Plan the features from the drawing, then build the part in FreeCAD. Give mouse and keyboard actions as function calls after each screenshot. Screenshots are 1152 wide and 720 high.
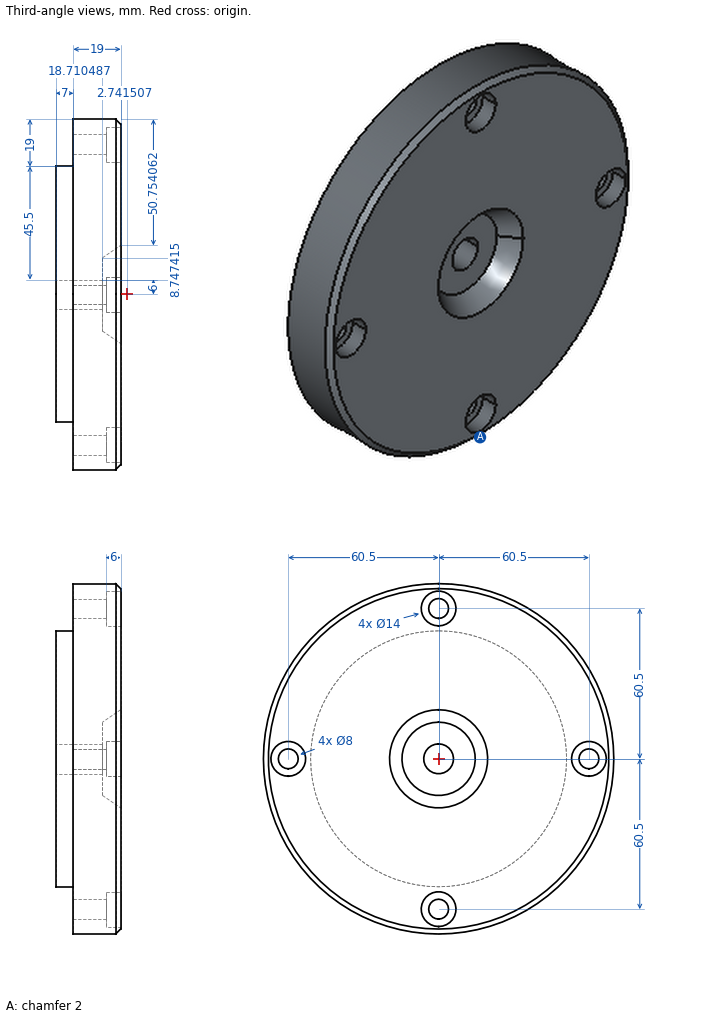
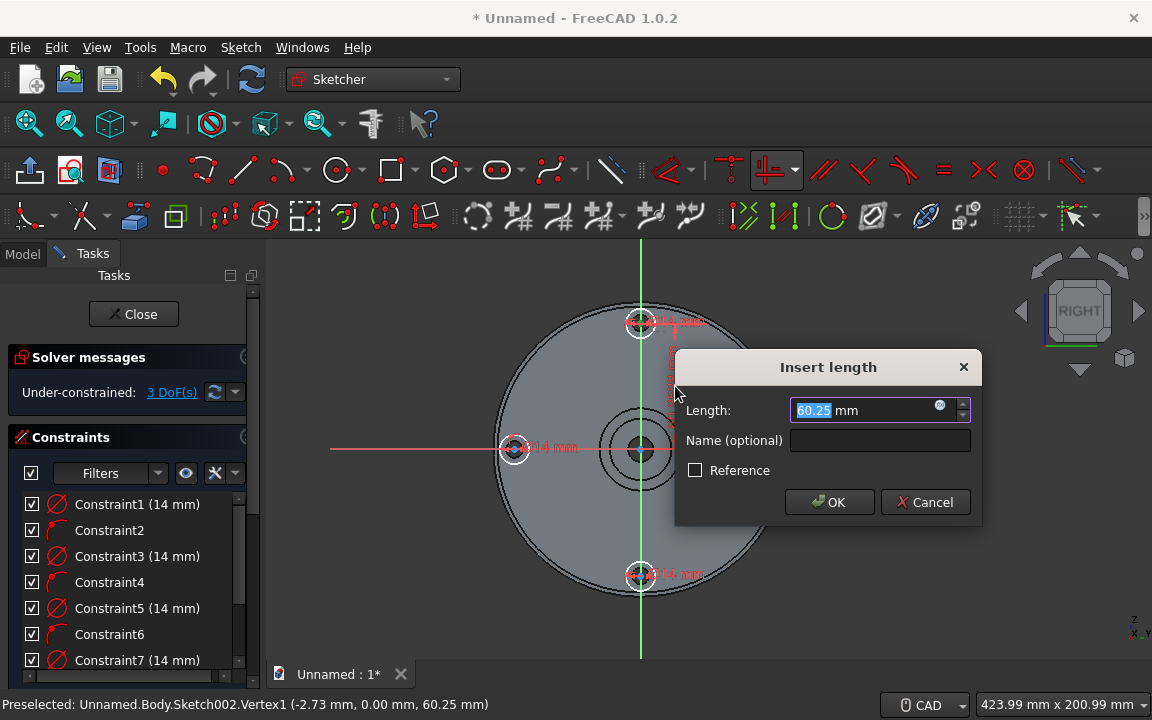
text(60.5)
key(Return)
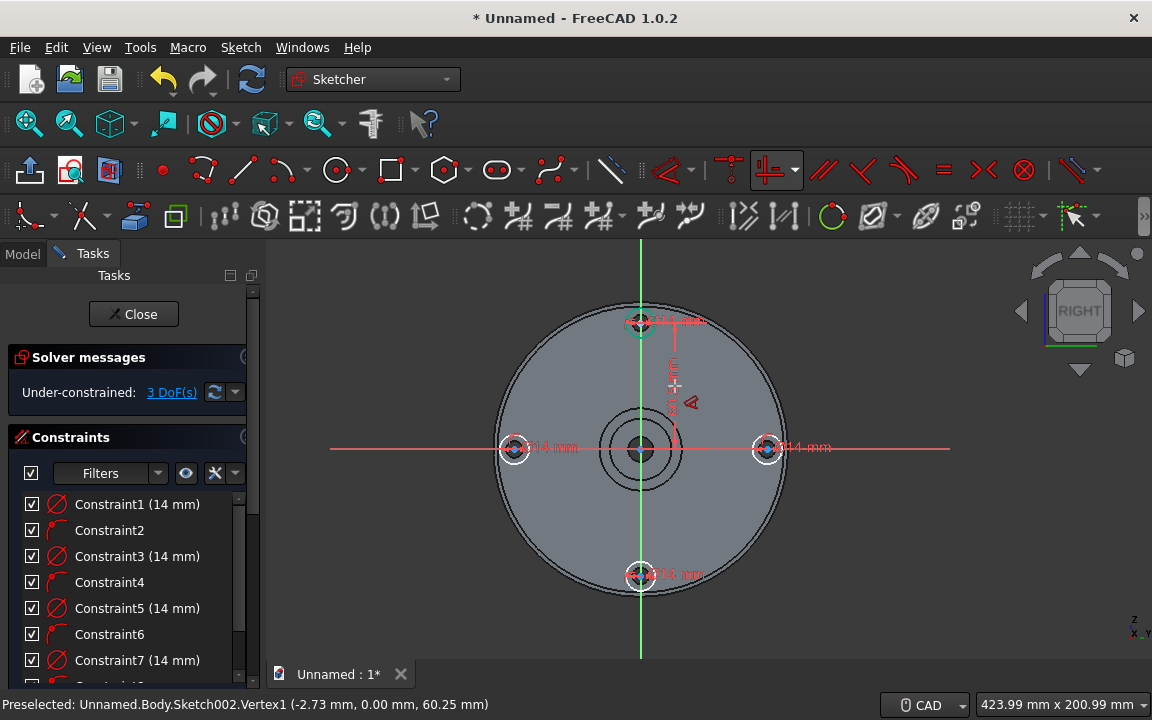
click(767, 449)
click(704, 483)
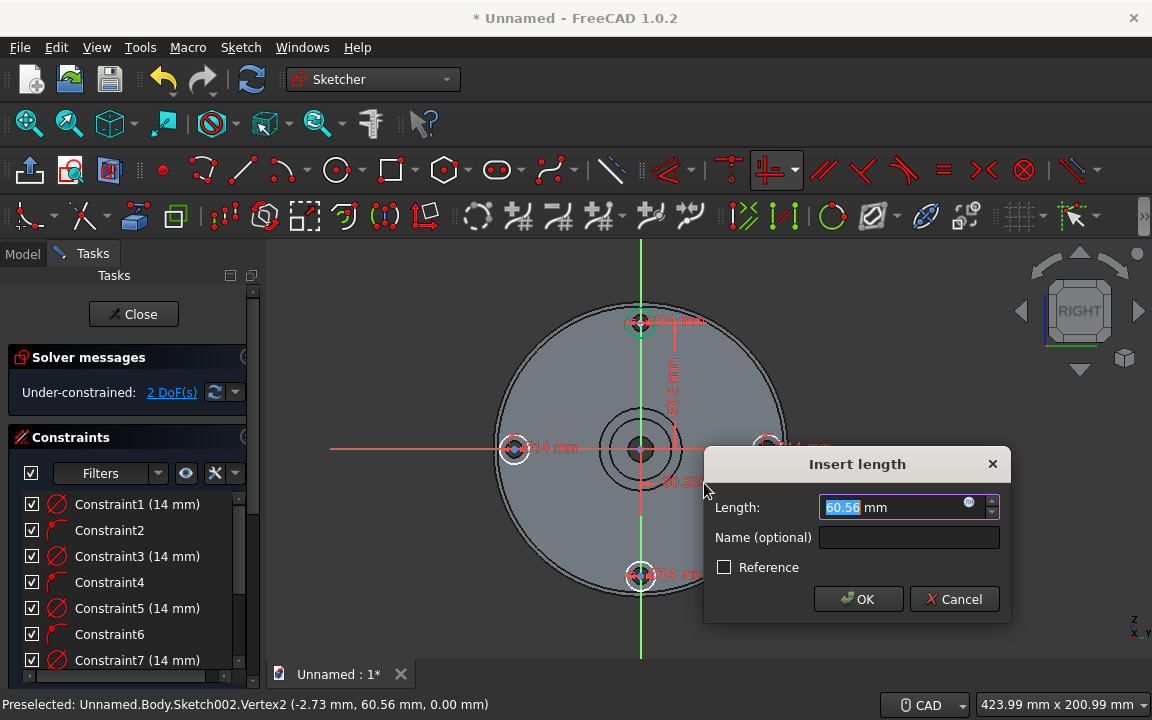
text(60.5)
key(Return)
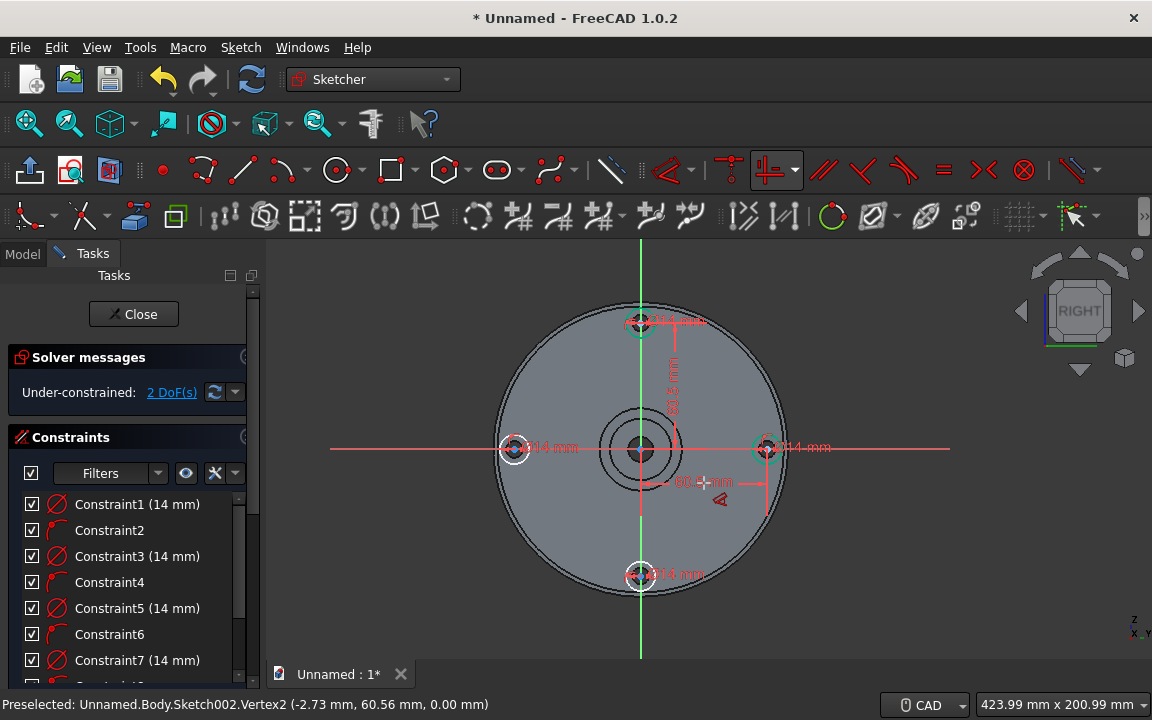
click(641, 576)
click(675, 513)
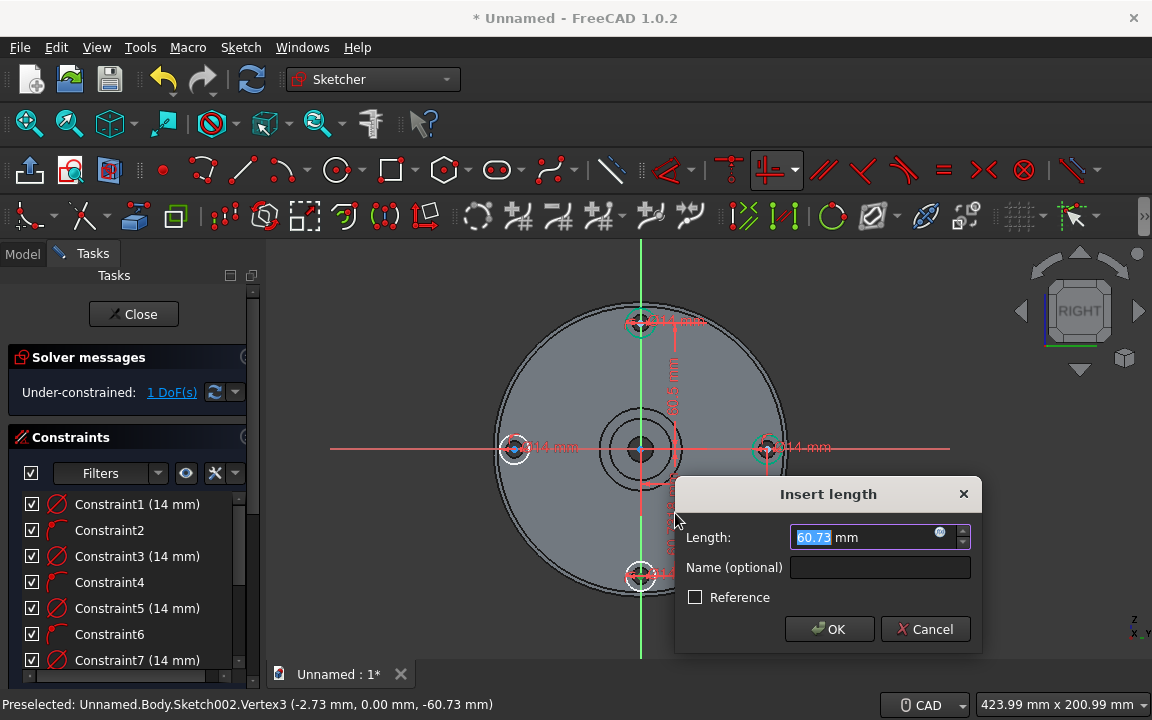
text(60.5)
key(Return)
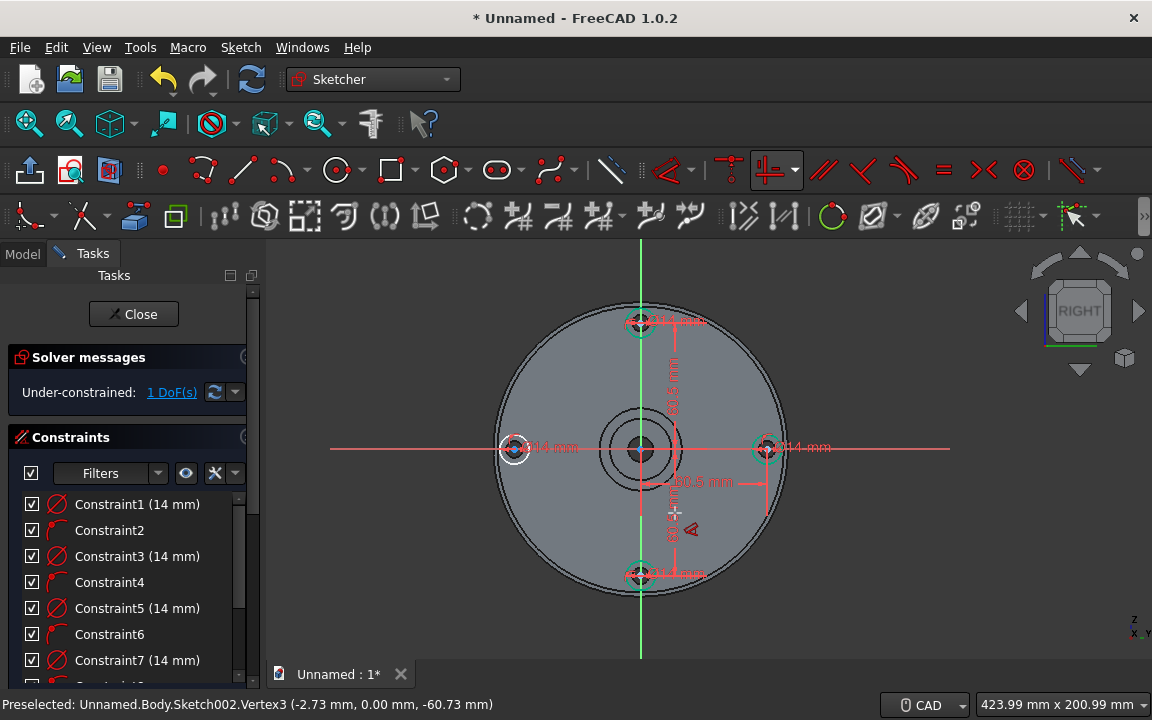
click(514, 449)
click(578, 483)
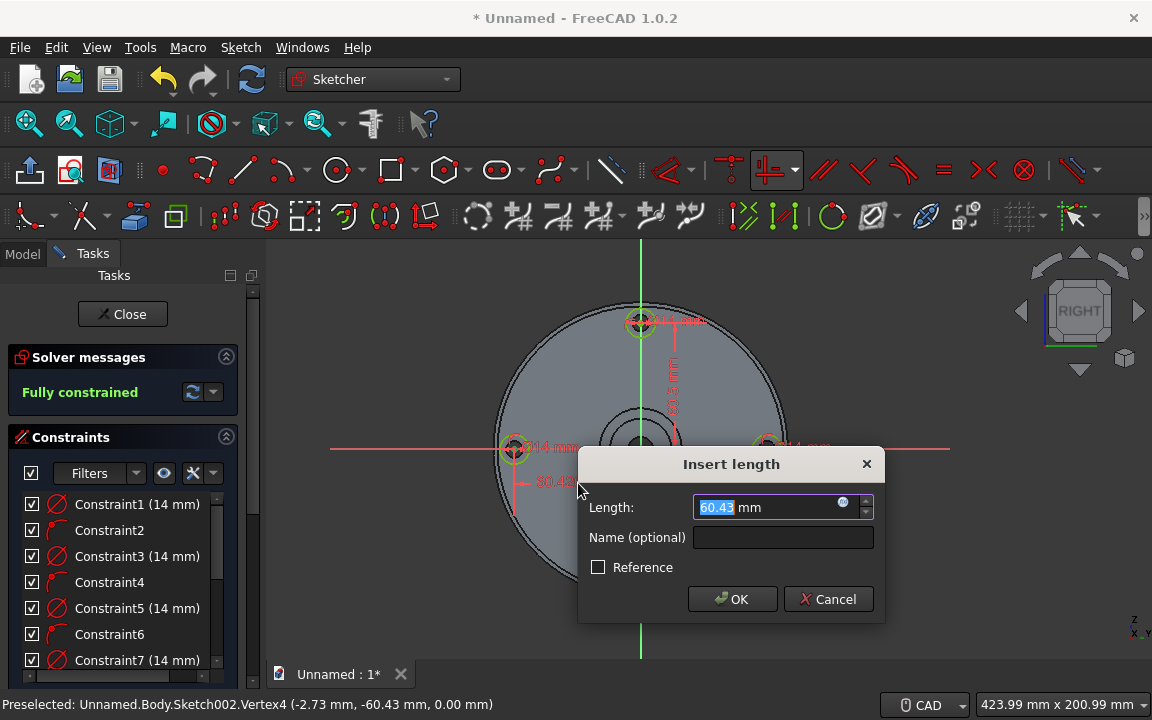
text(60.5)
key(Return)
key(Escape)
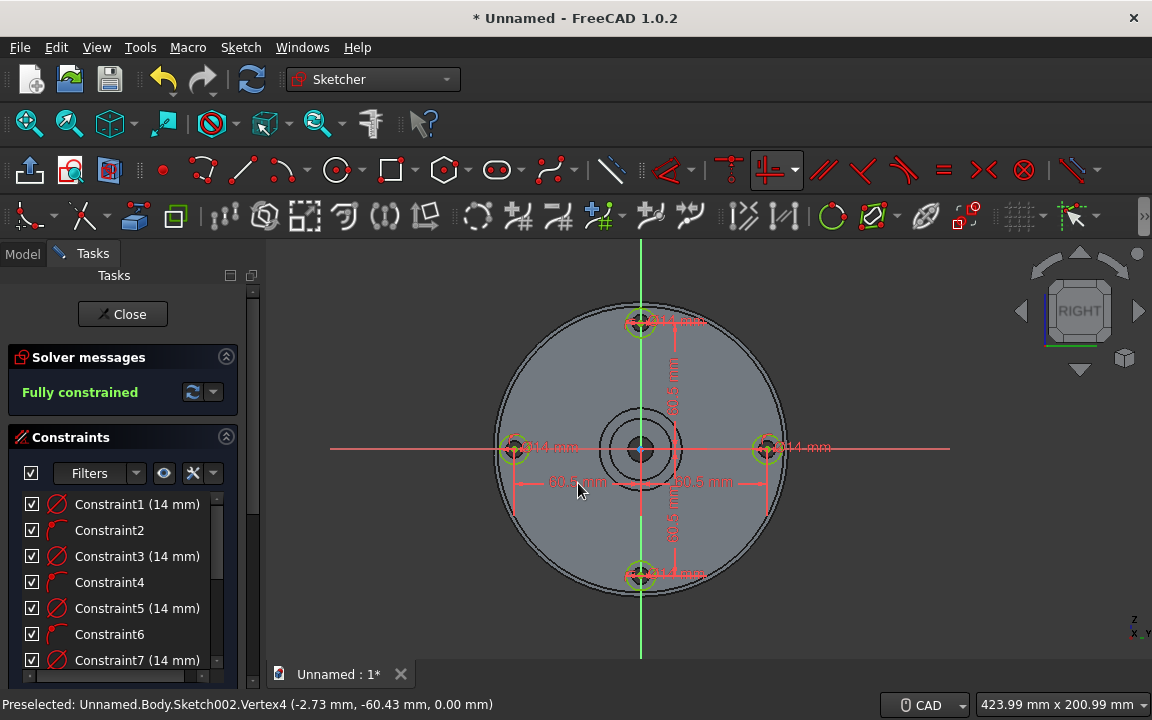
click(123, 314)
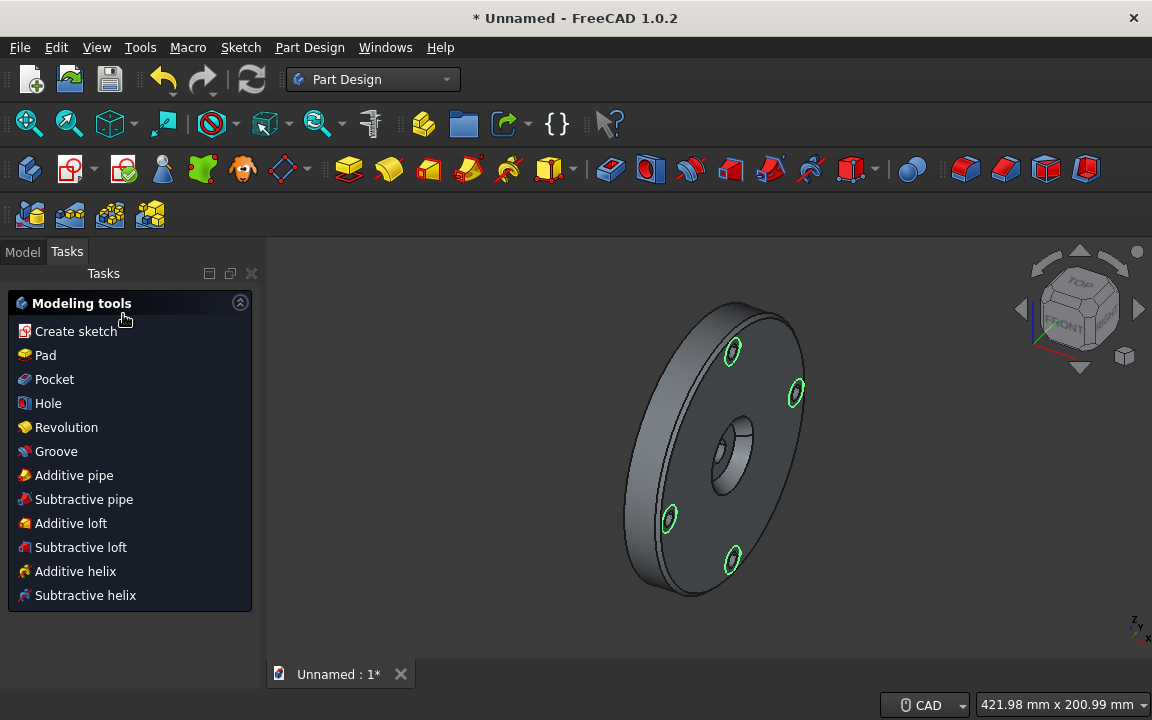
click(612, 170)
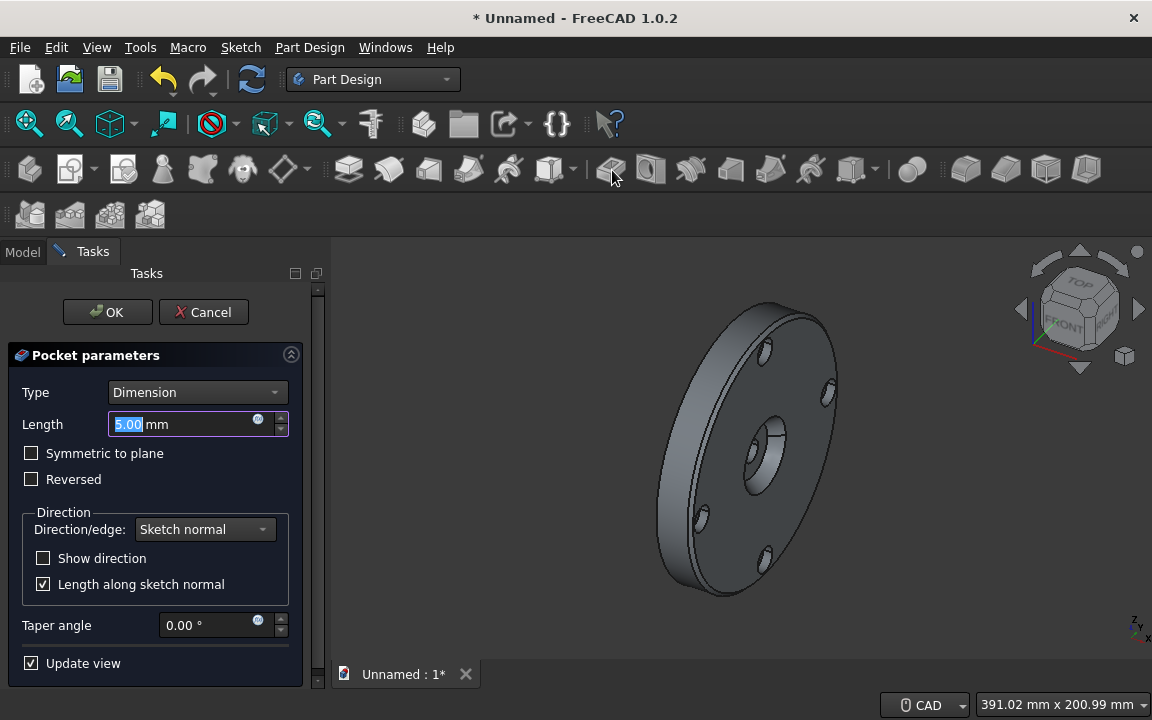
text(6)
key(Tab)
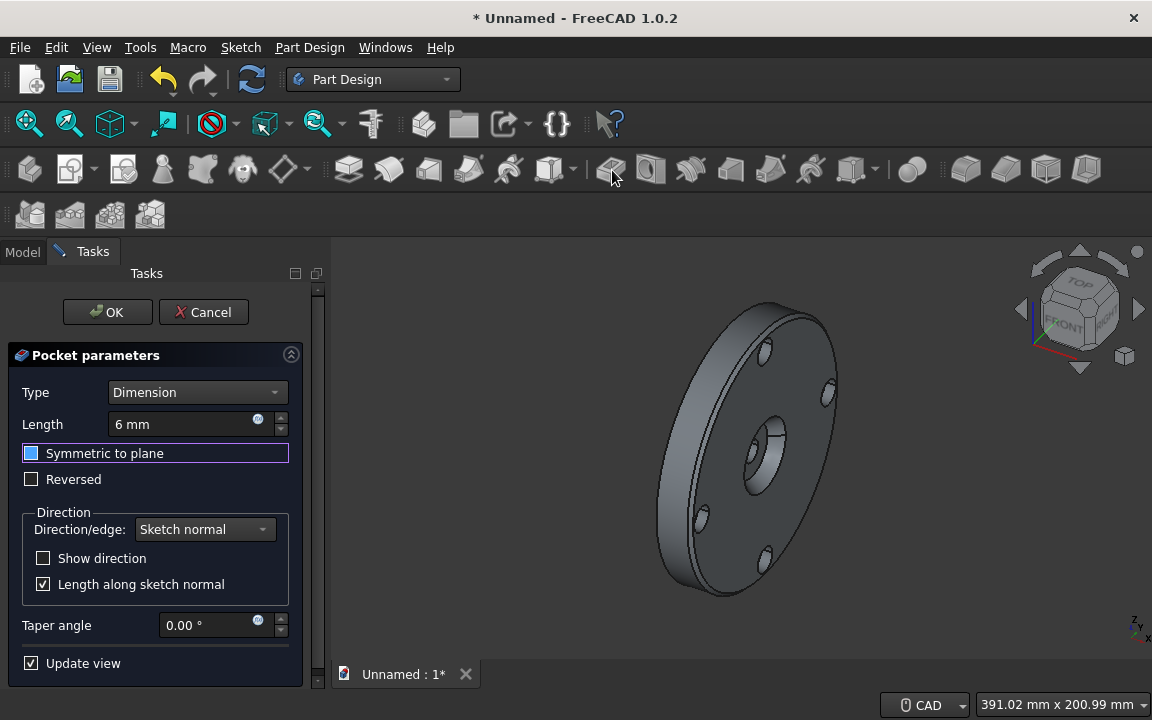
click(108, 312)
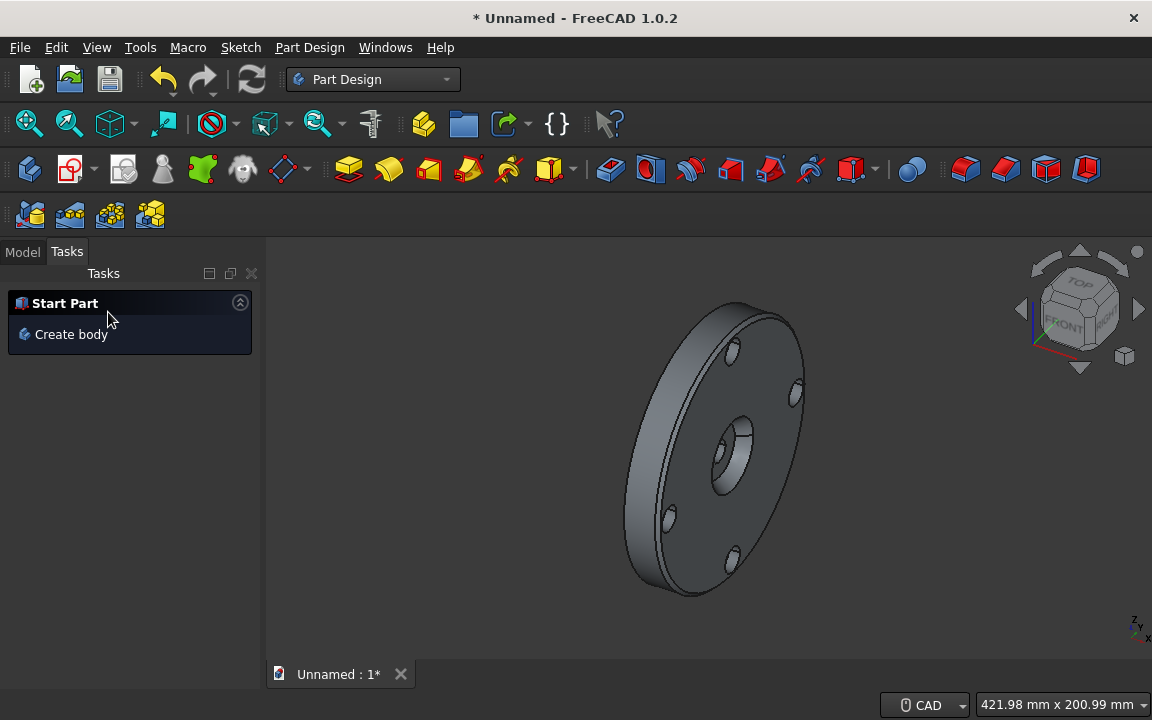
key(0)